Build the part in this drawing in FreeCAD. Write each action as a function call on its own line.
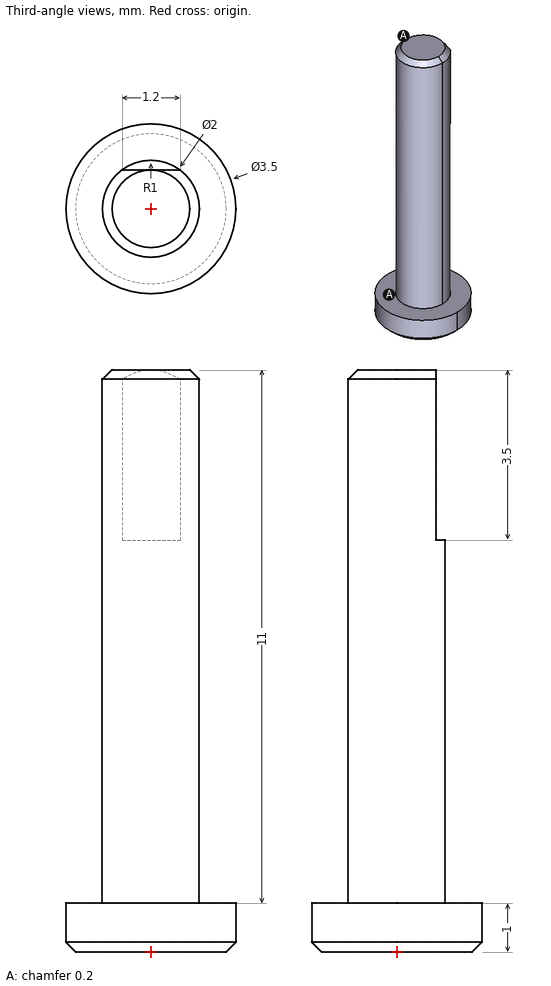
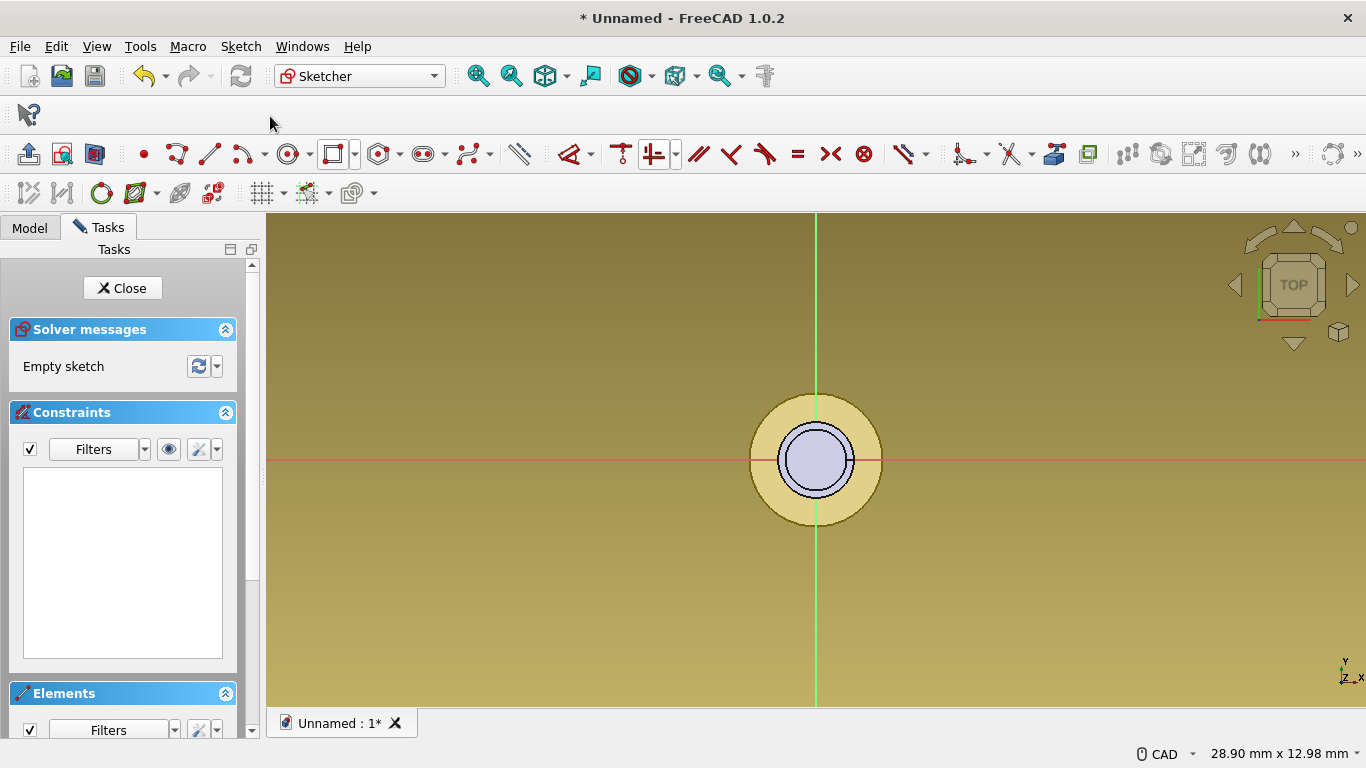
click(95, 154)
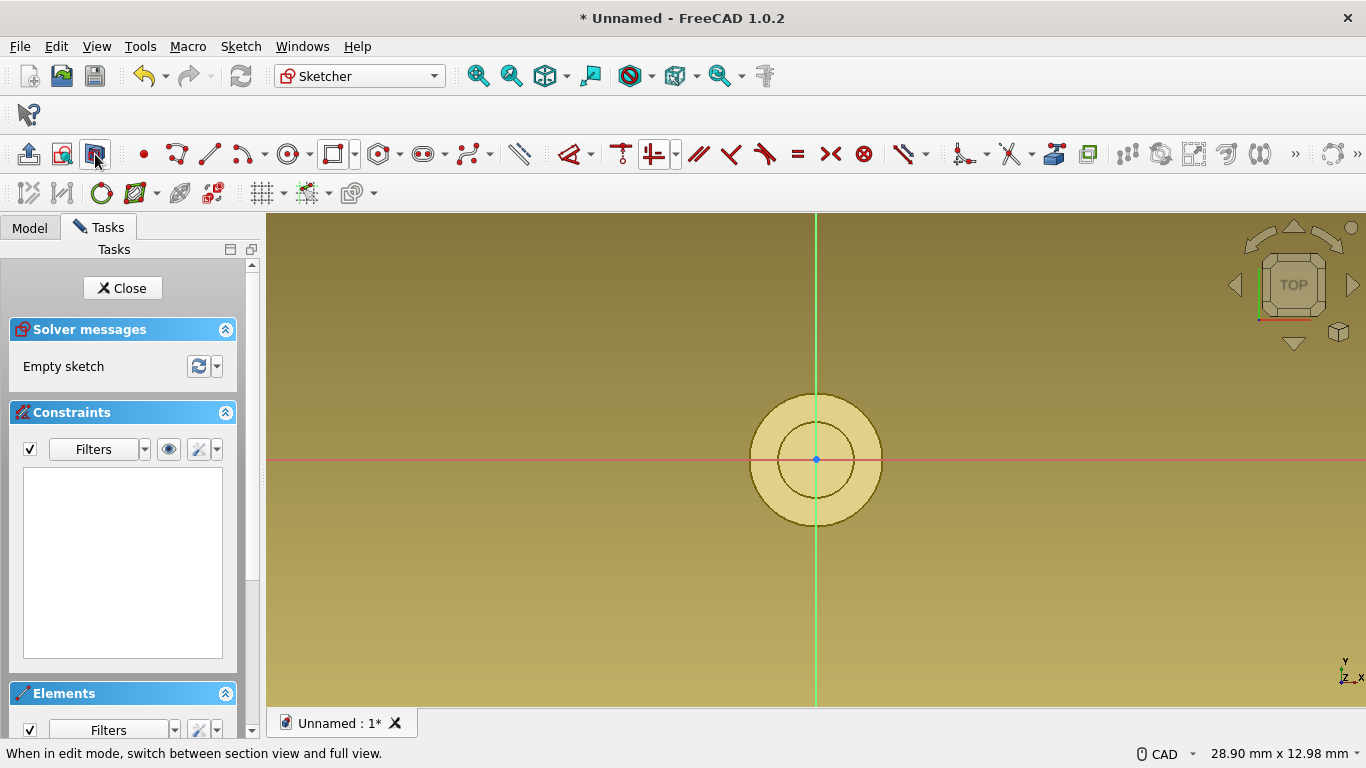
scroll(827, 438, up, 10)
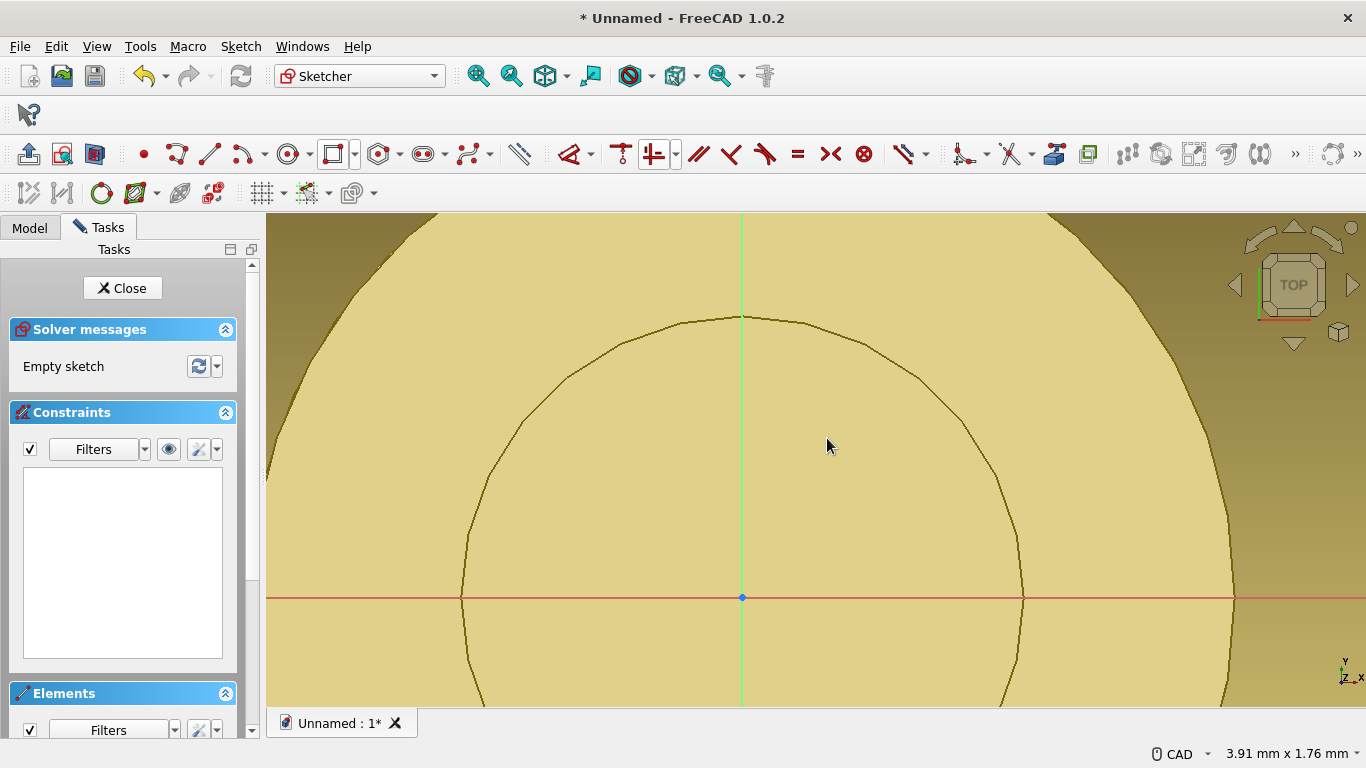
key(g)
key(l)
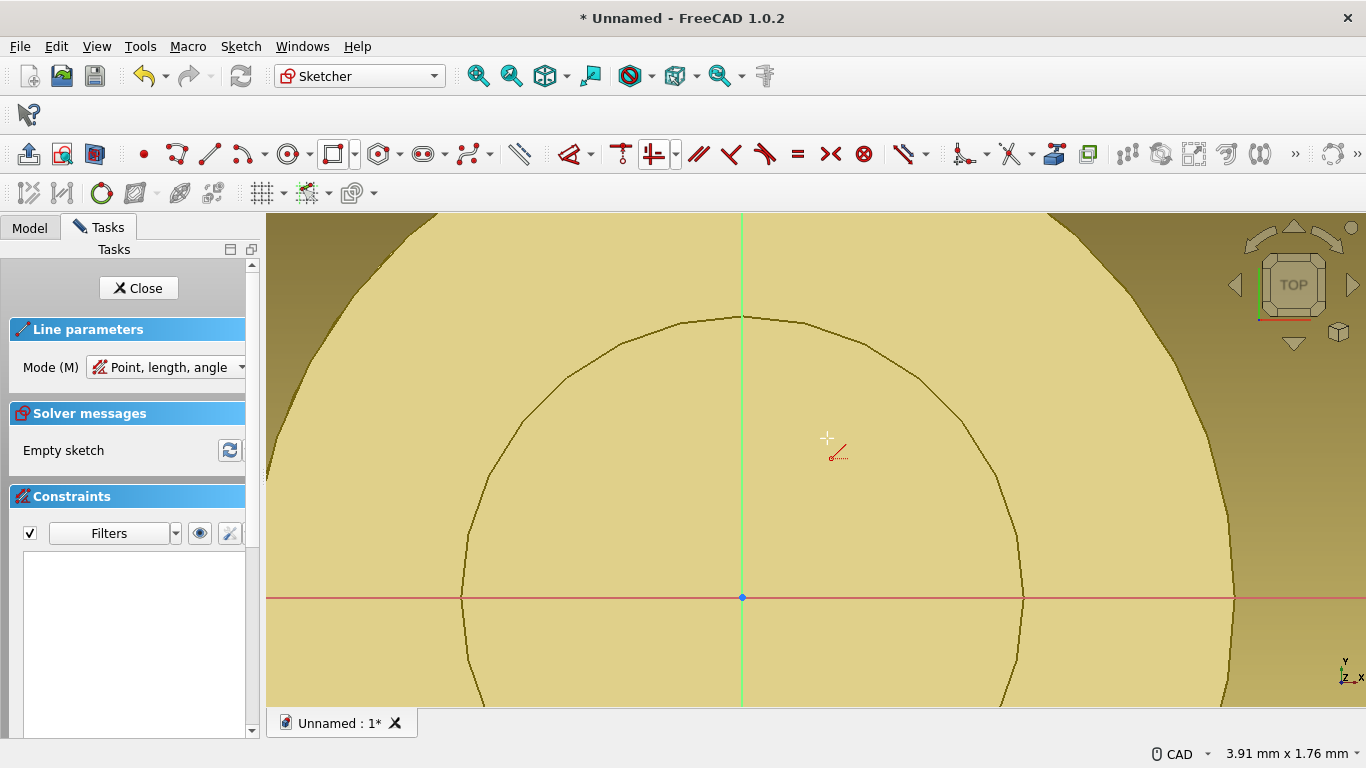
click(574, 373)
click(911, 373)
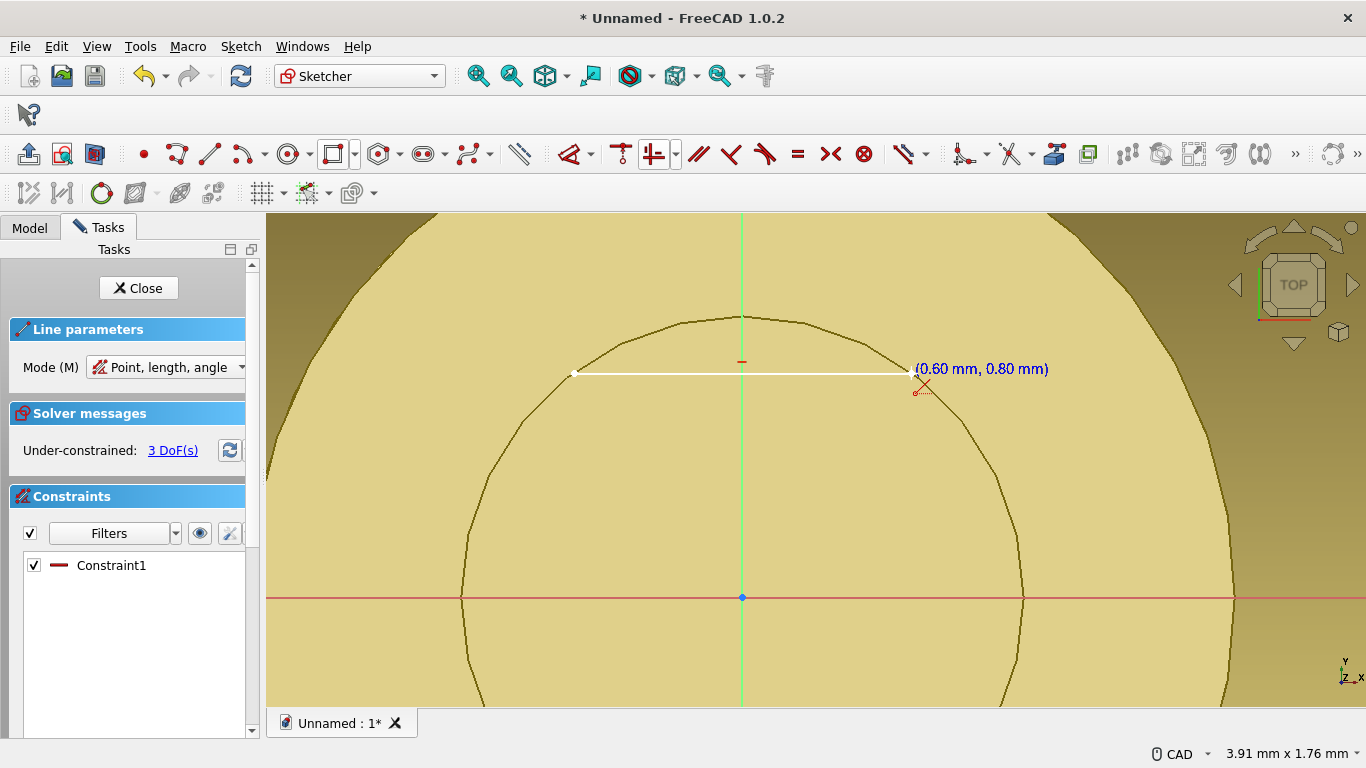
key(g)
key(3)
key(a)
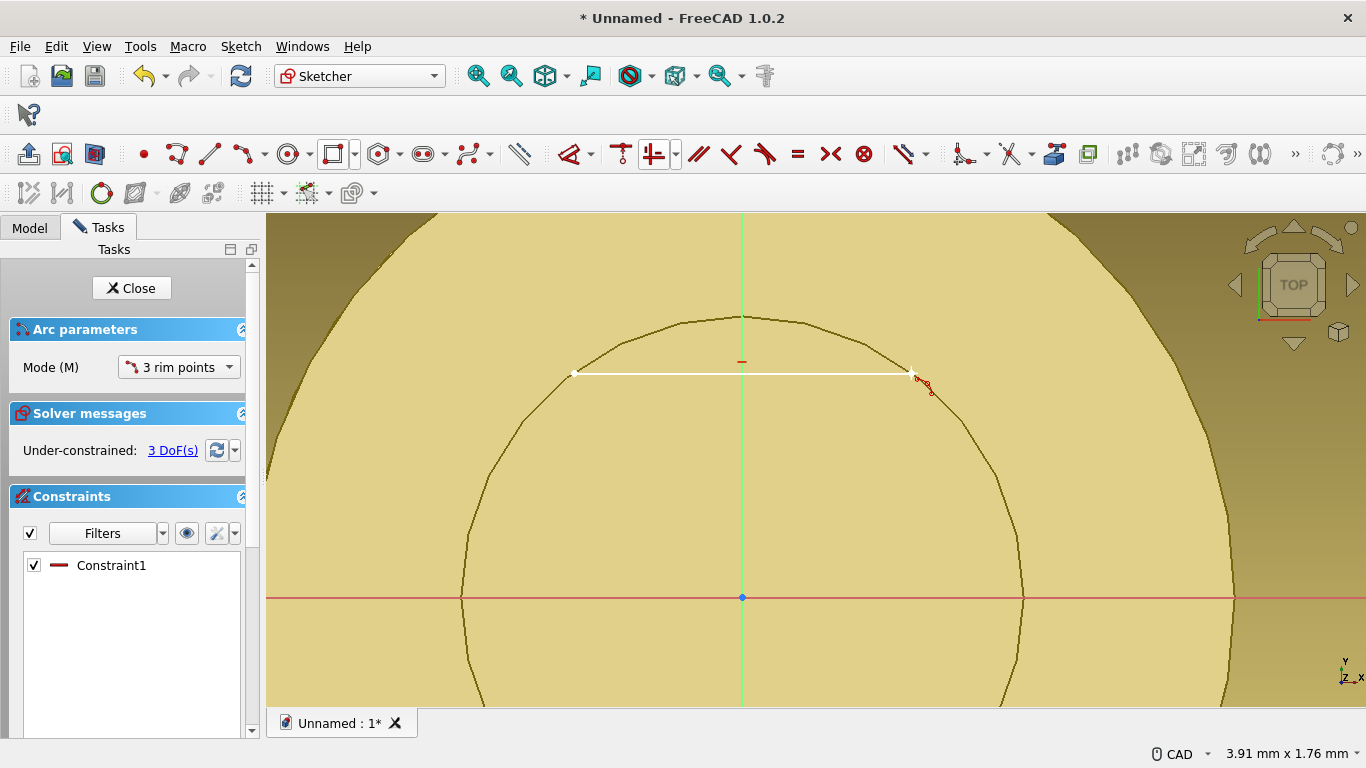
click(911, 374)
click(574, 374)
click(779, 319)
key(Escape)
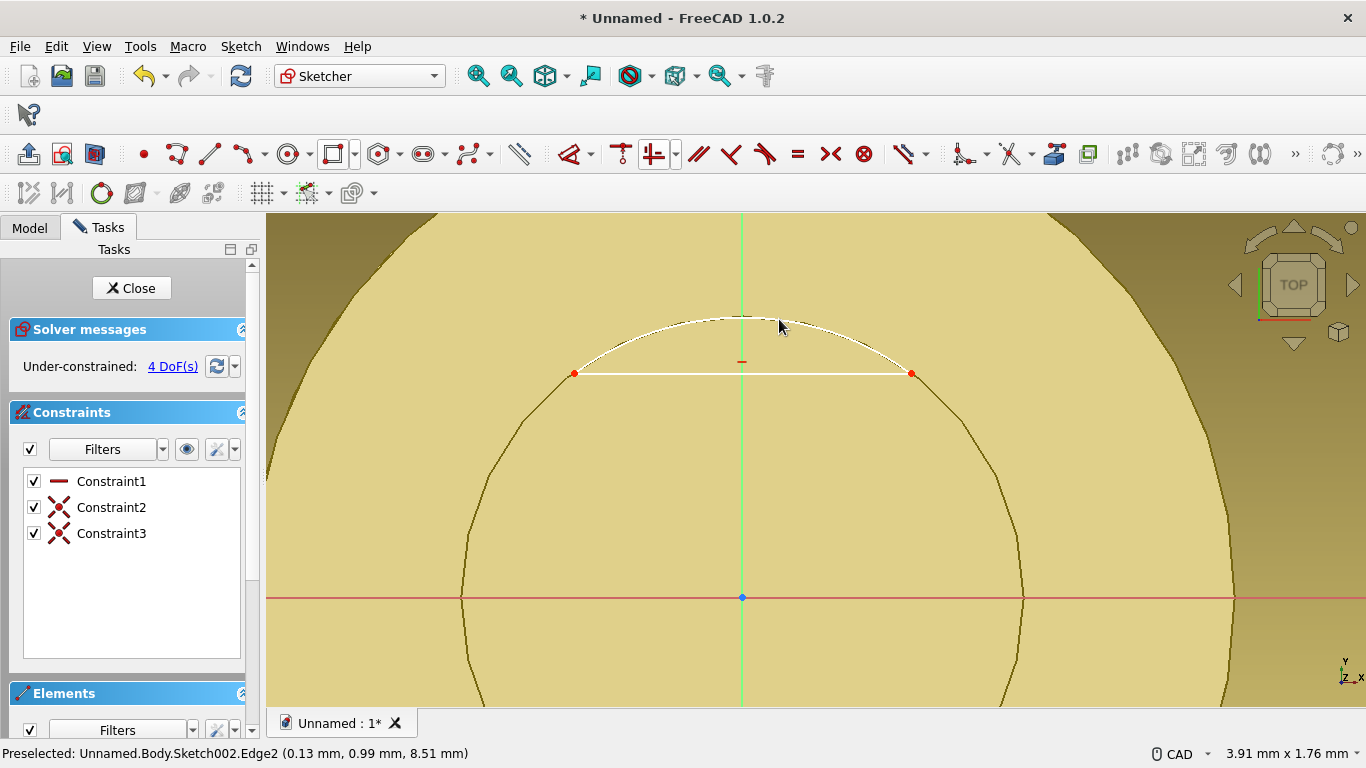
drag(732, 588, 752, 608)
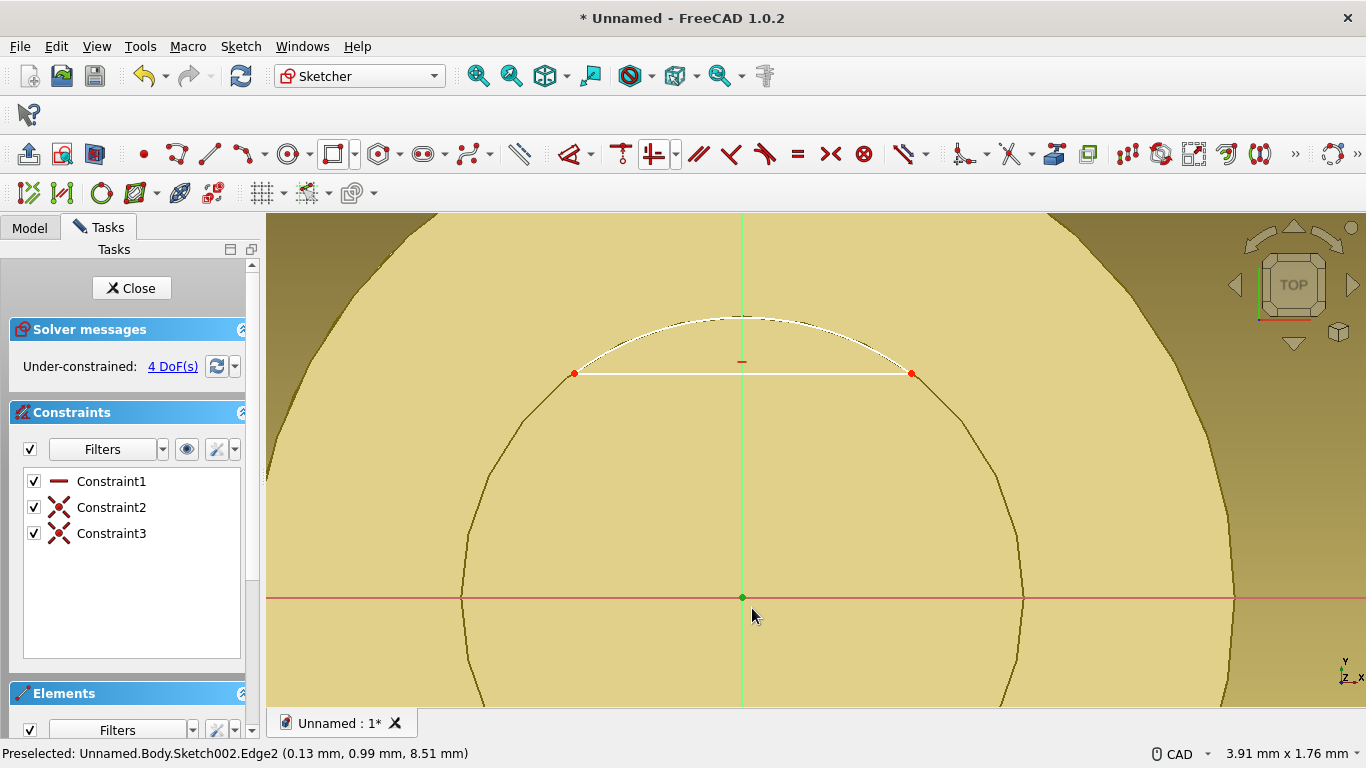
click(621, 154)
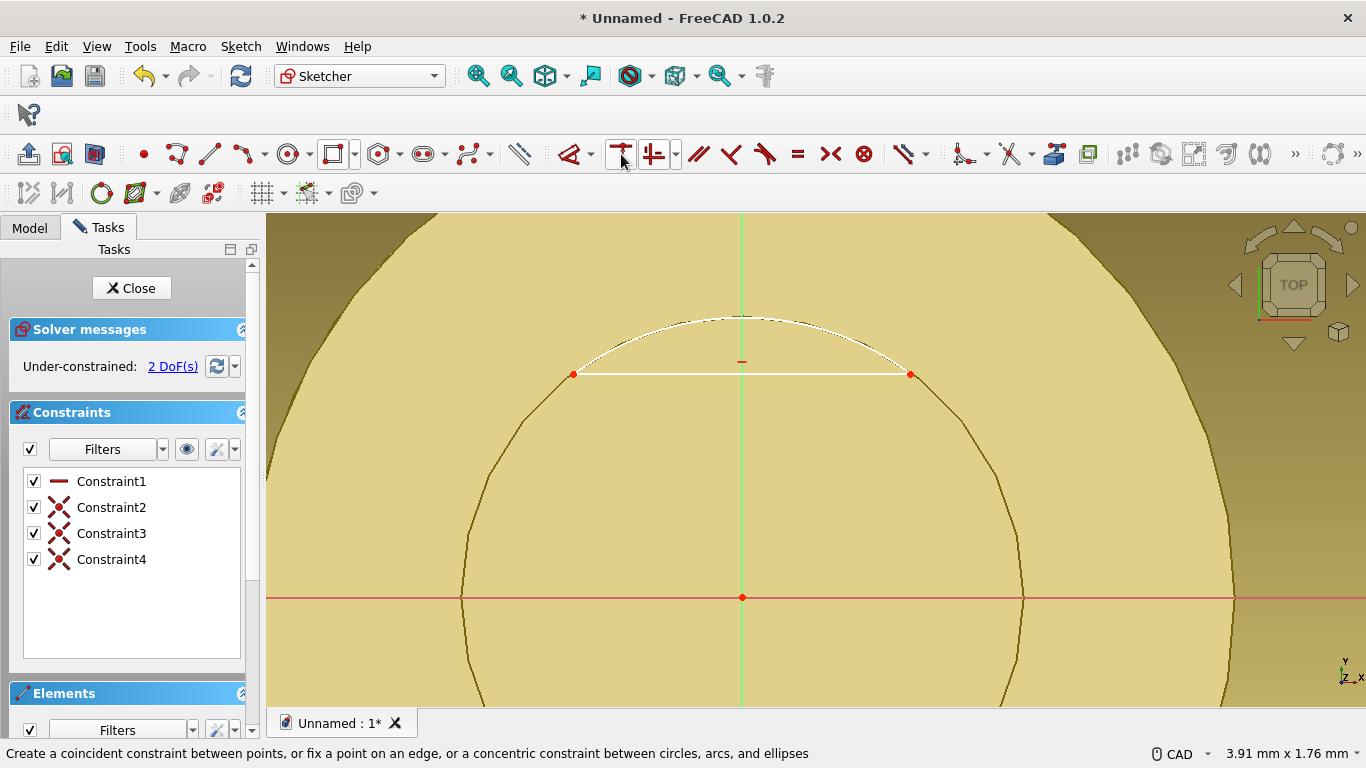
click(568, 154)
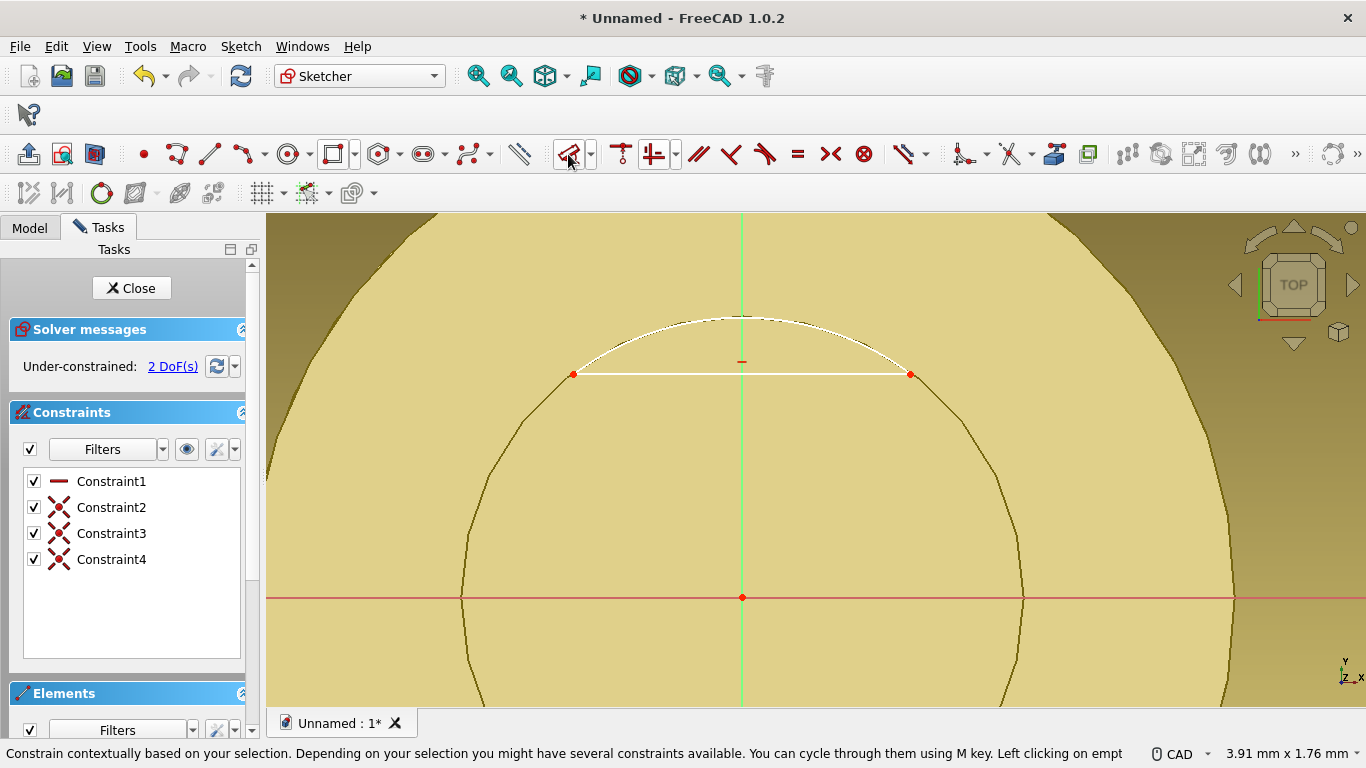
click(814, 327)
click(822, 296)